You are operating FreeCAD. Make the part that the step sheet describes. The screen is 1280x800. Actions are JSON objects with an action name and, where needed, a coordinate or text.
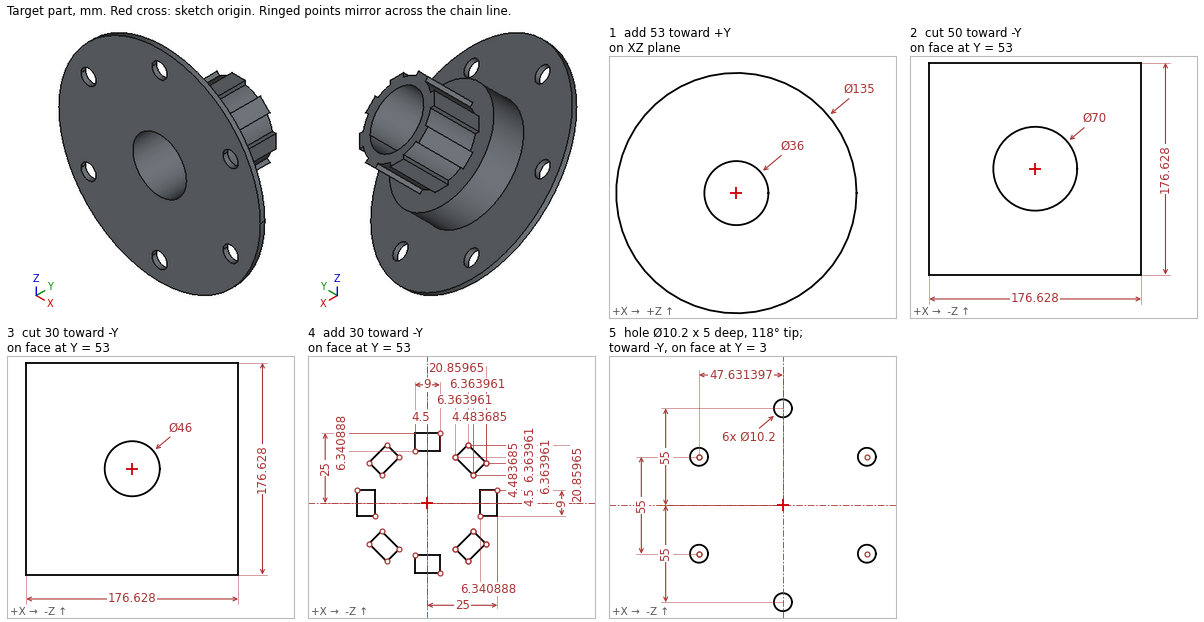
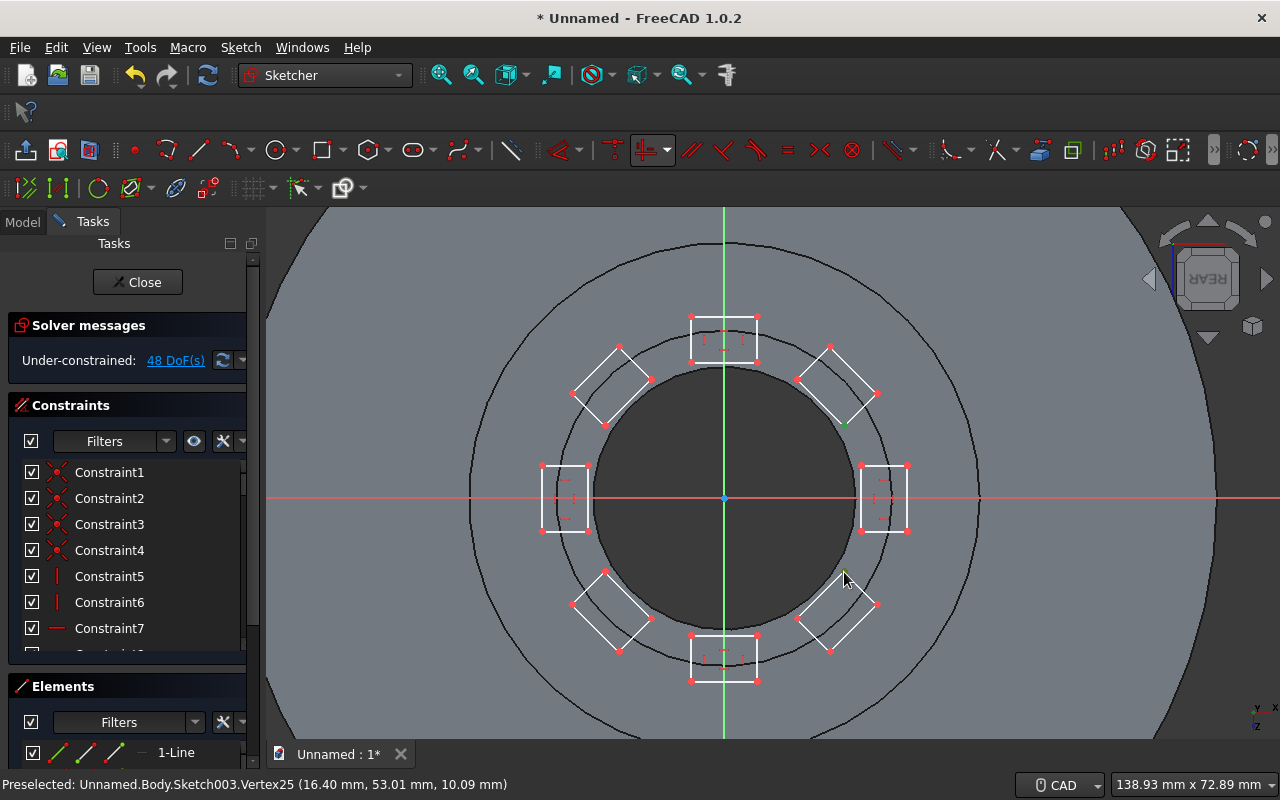
{"action": "left_click", "coordinate": [353, 498]}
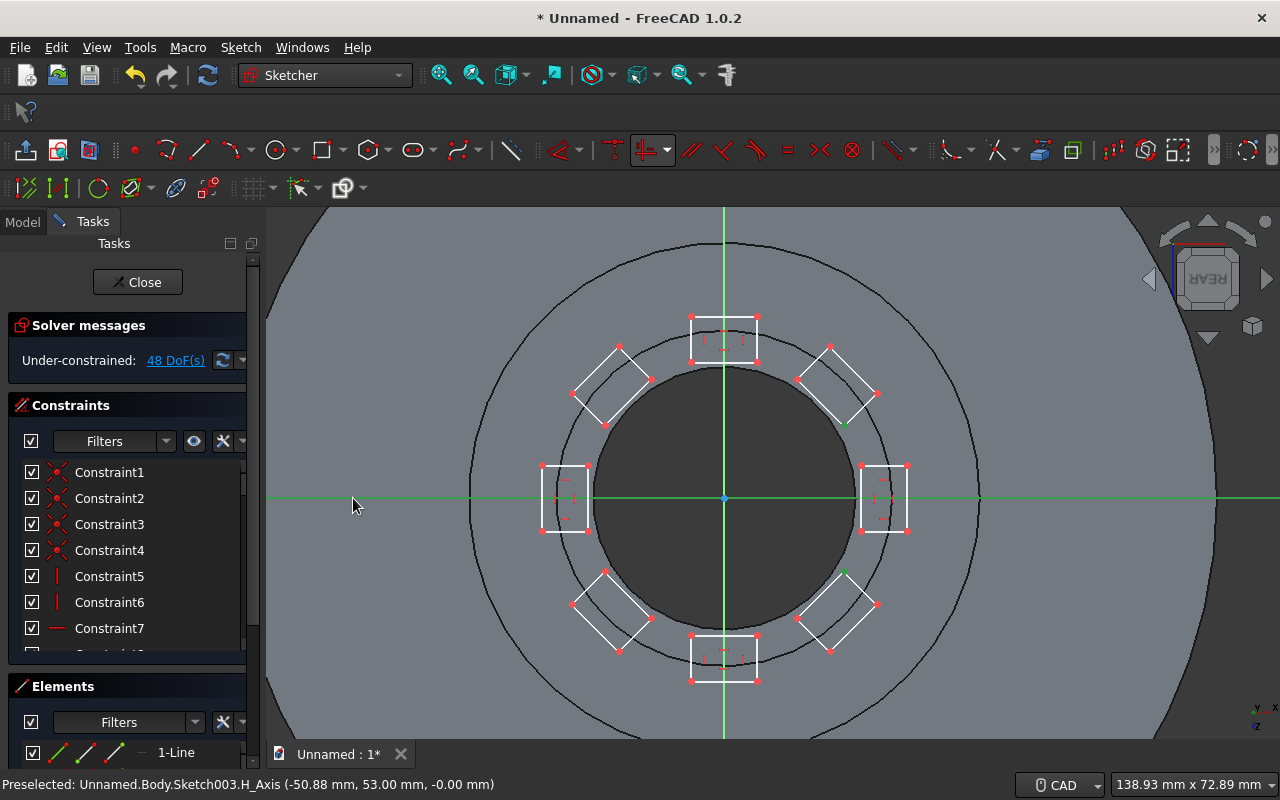
{"action": "left_click", "coordinate": [820, 150]}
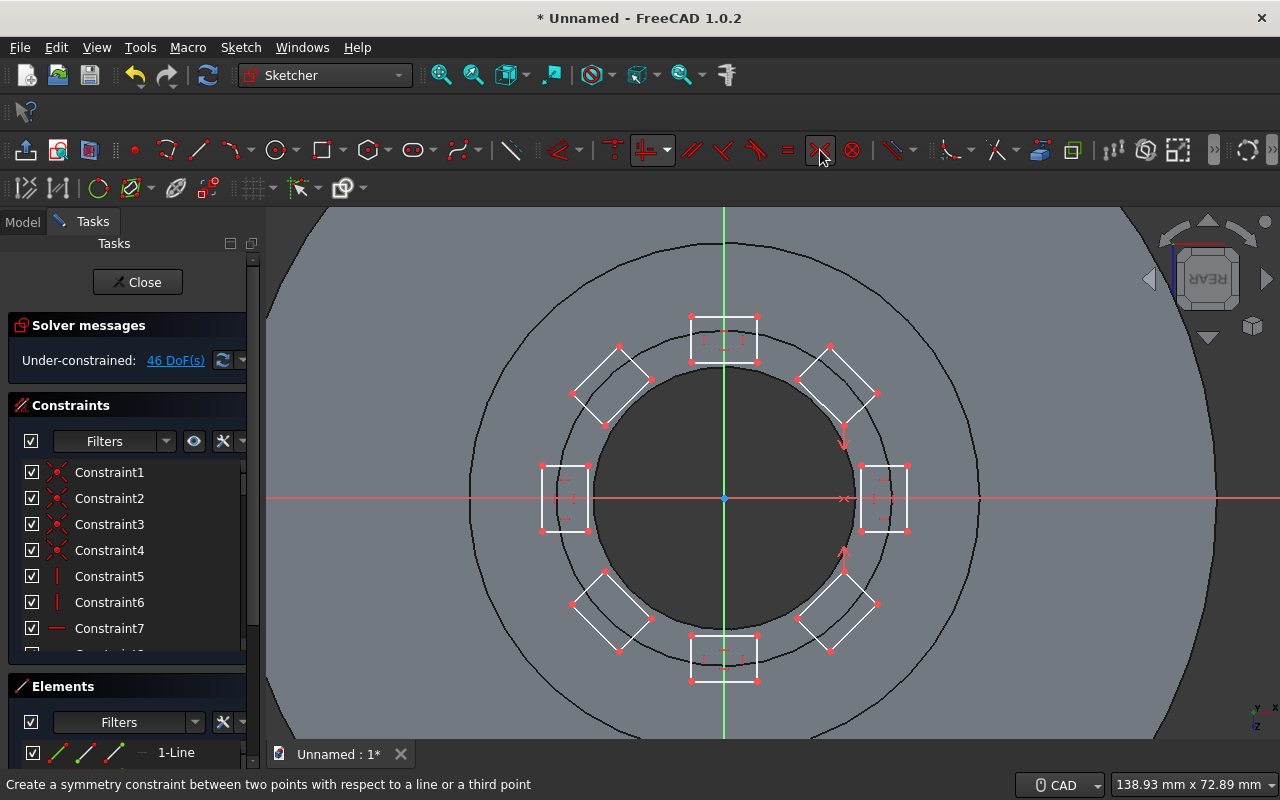
{"action": "left_click", "coordinate": [797, 380]}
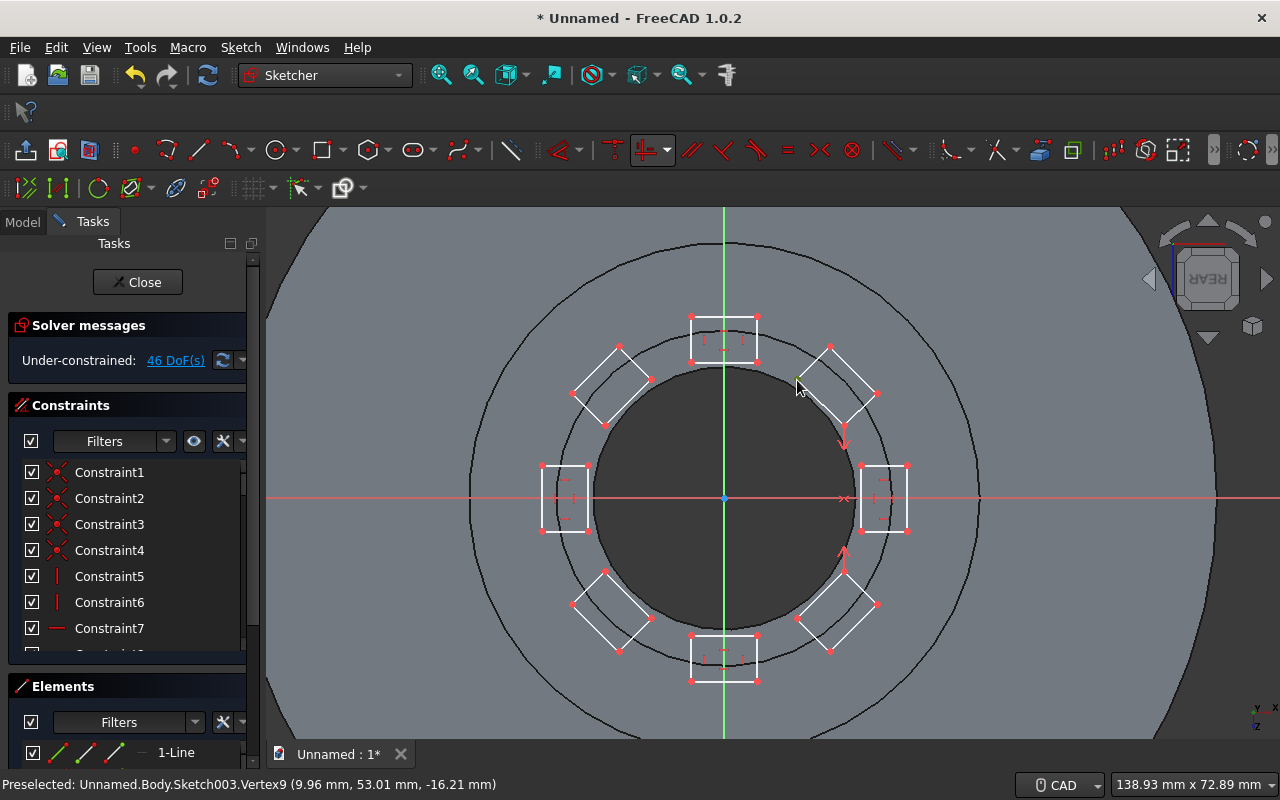
{"action": "left_click", "coordinate": [797, 619]}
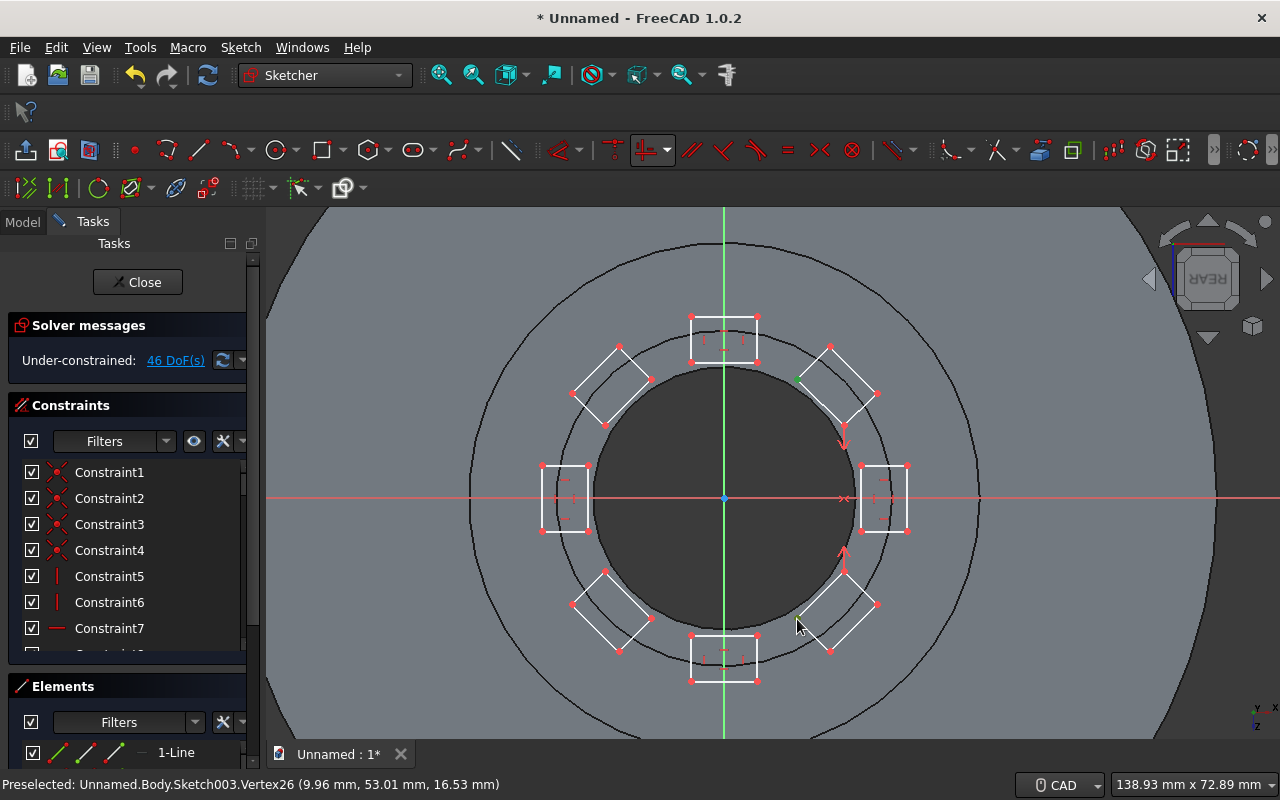
{"action": "left_click", "coordinate": [353, 498]}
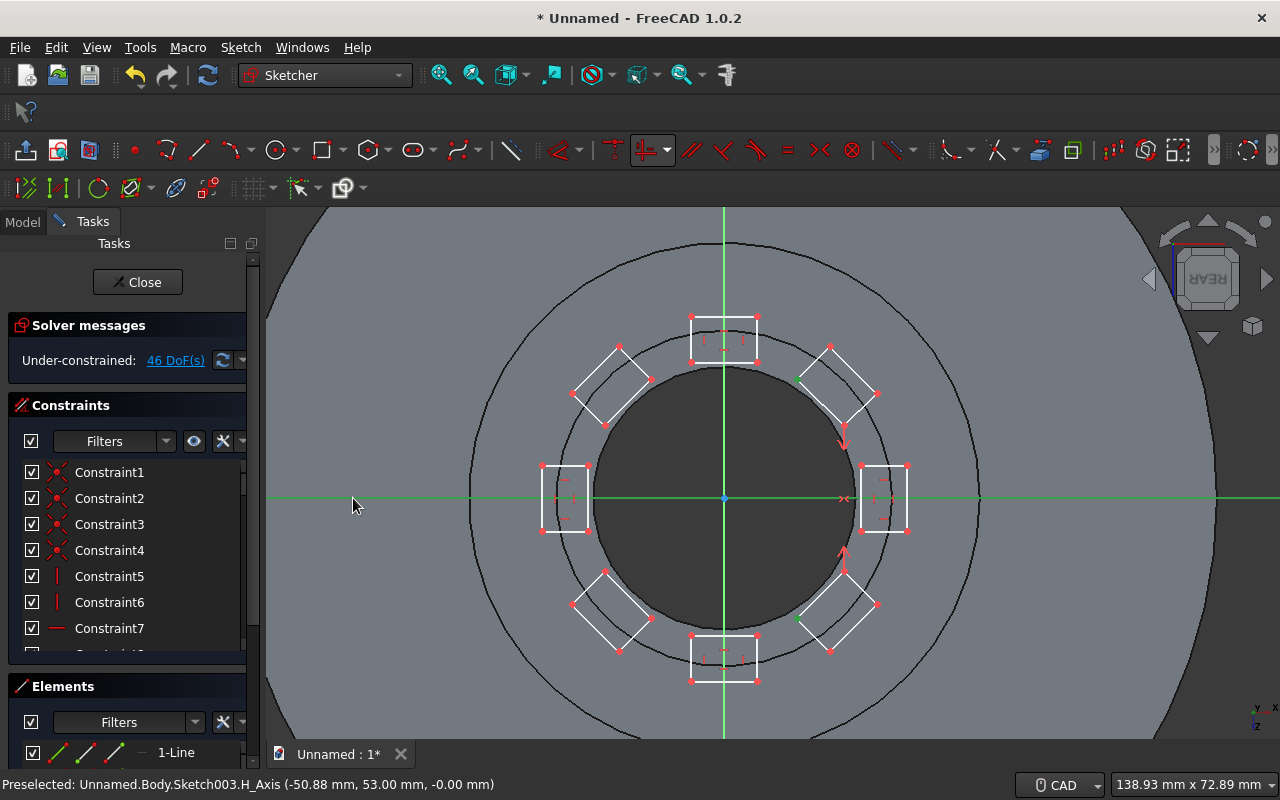
{"action": "left_click", "coordinate": [820, 150]}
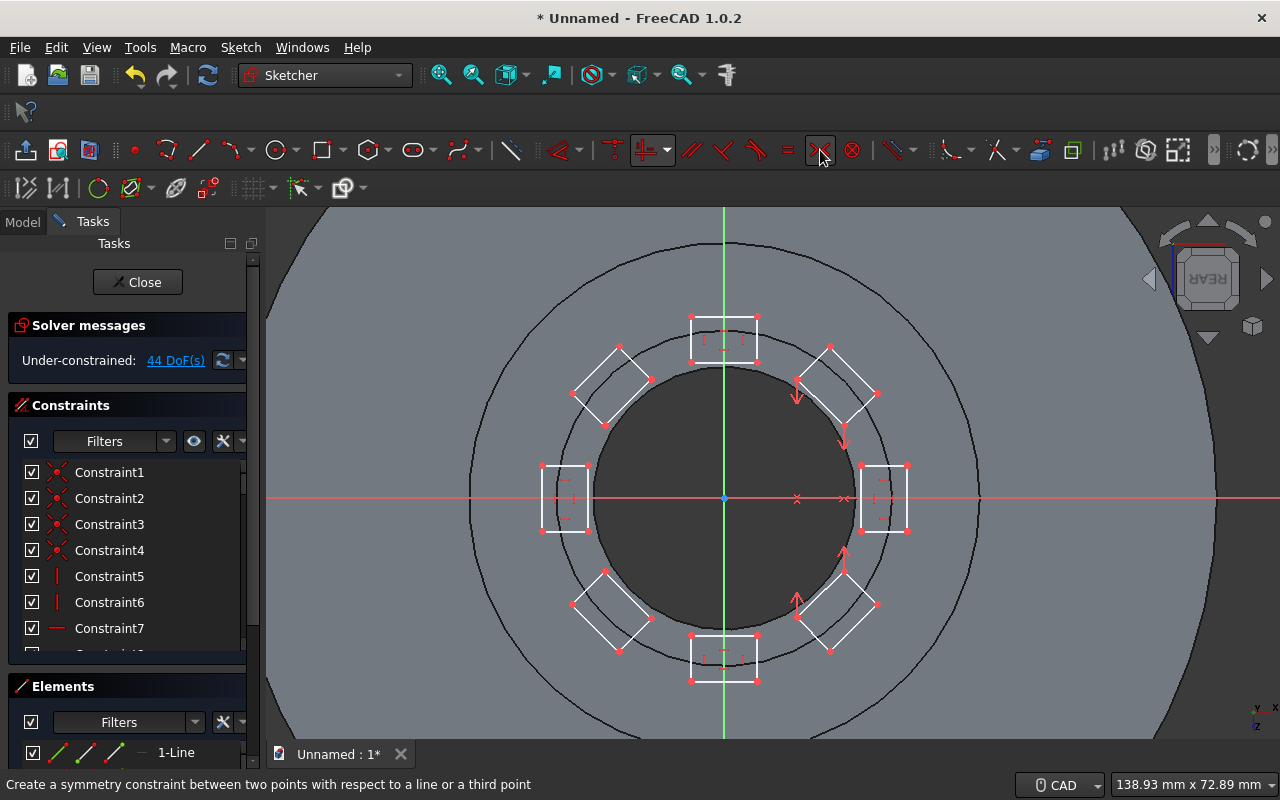
{"action": "left_click", "coordinate": [830, 347]}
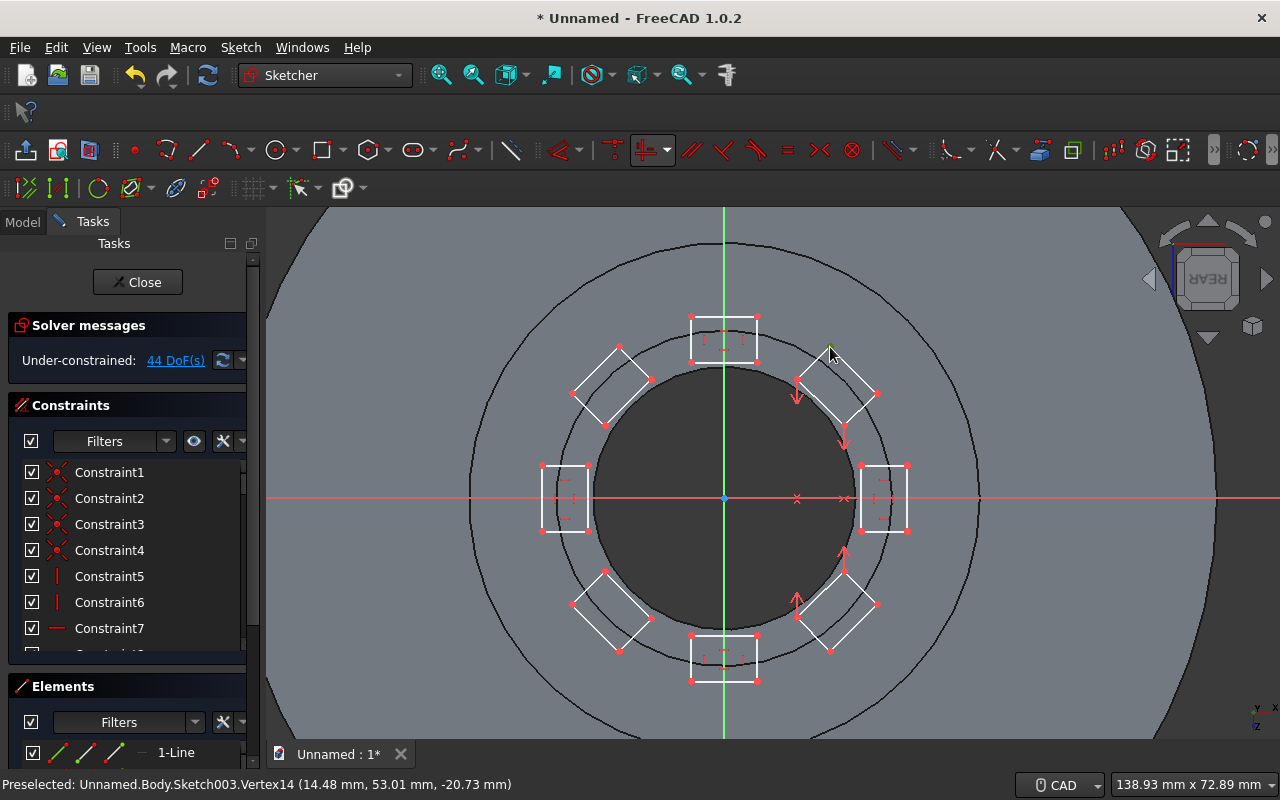
{"action": "left_click", "coordinate": [830, 652]}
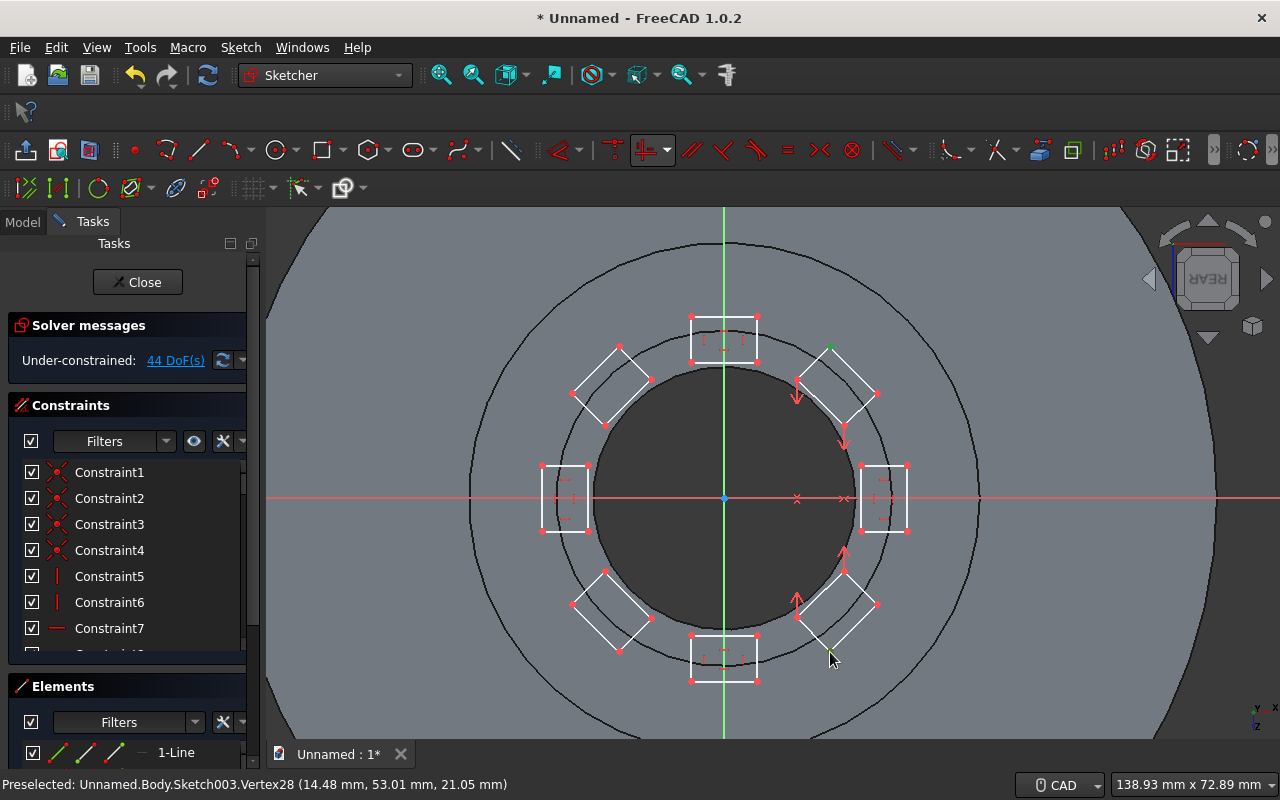
{"action": "left_click", "coordinate": [353, 498]}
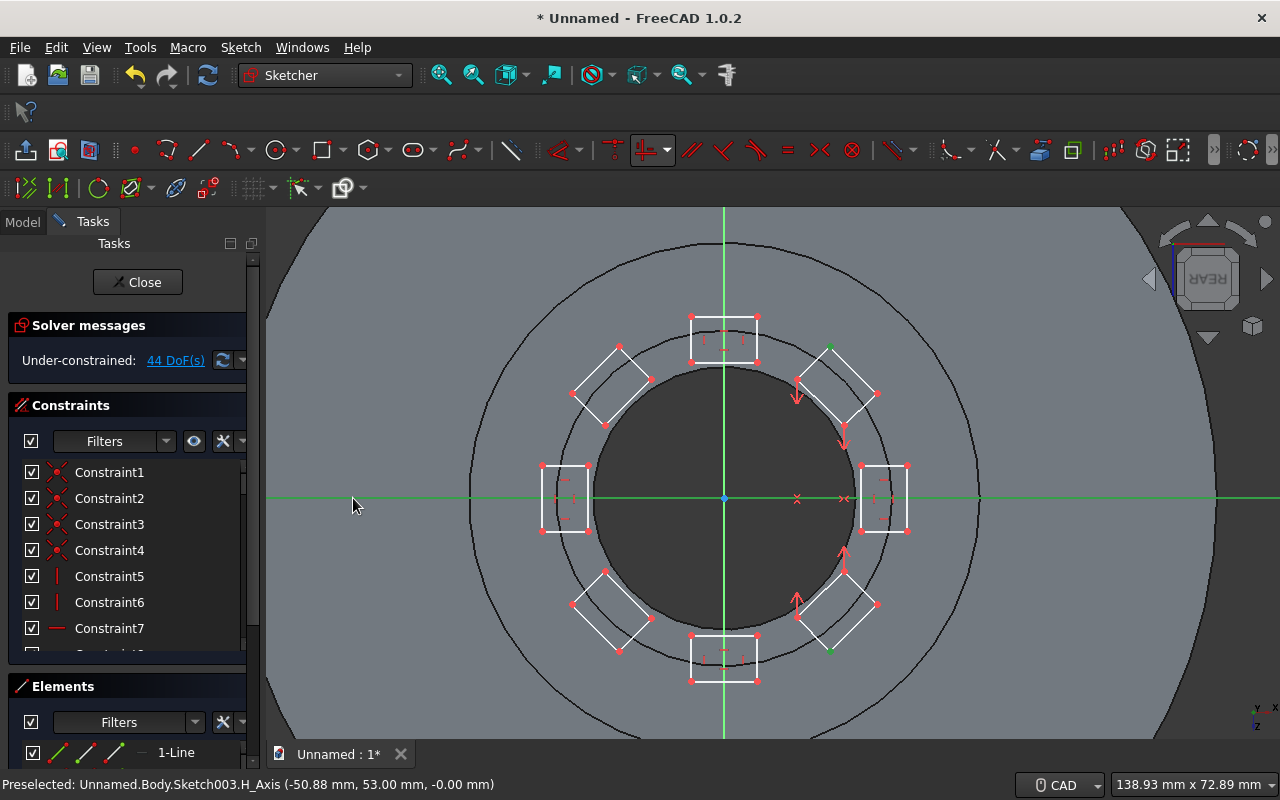
{"action": "left_click", "coordinate": [820, 150]}